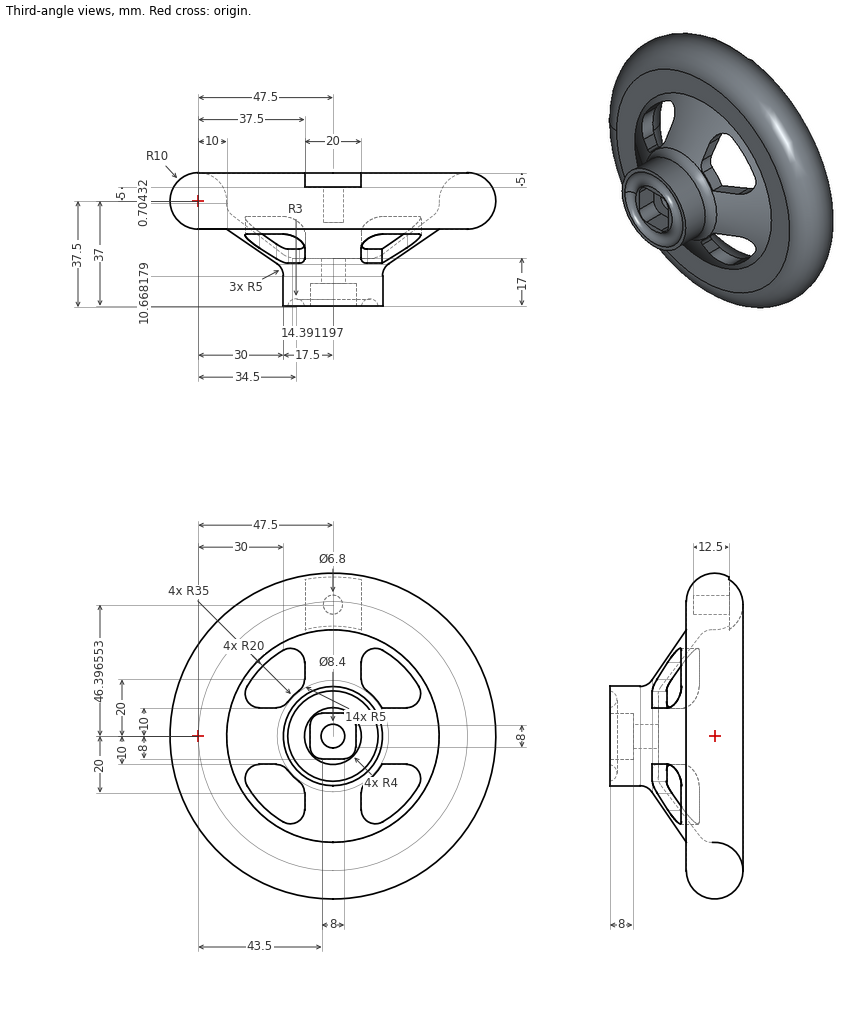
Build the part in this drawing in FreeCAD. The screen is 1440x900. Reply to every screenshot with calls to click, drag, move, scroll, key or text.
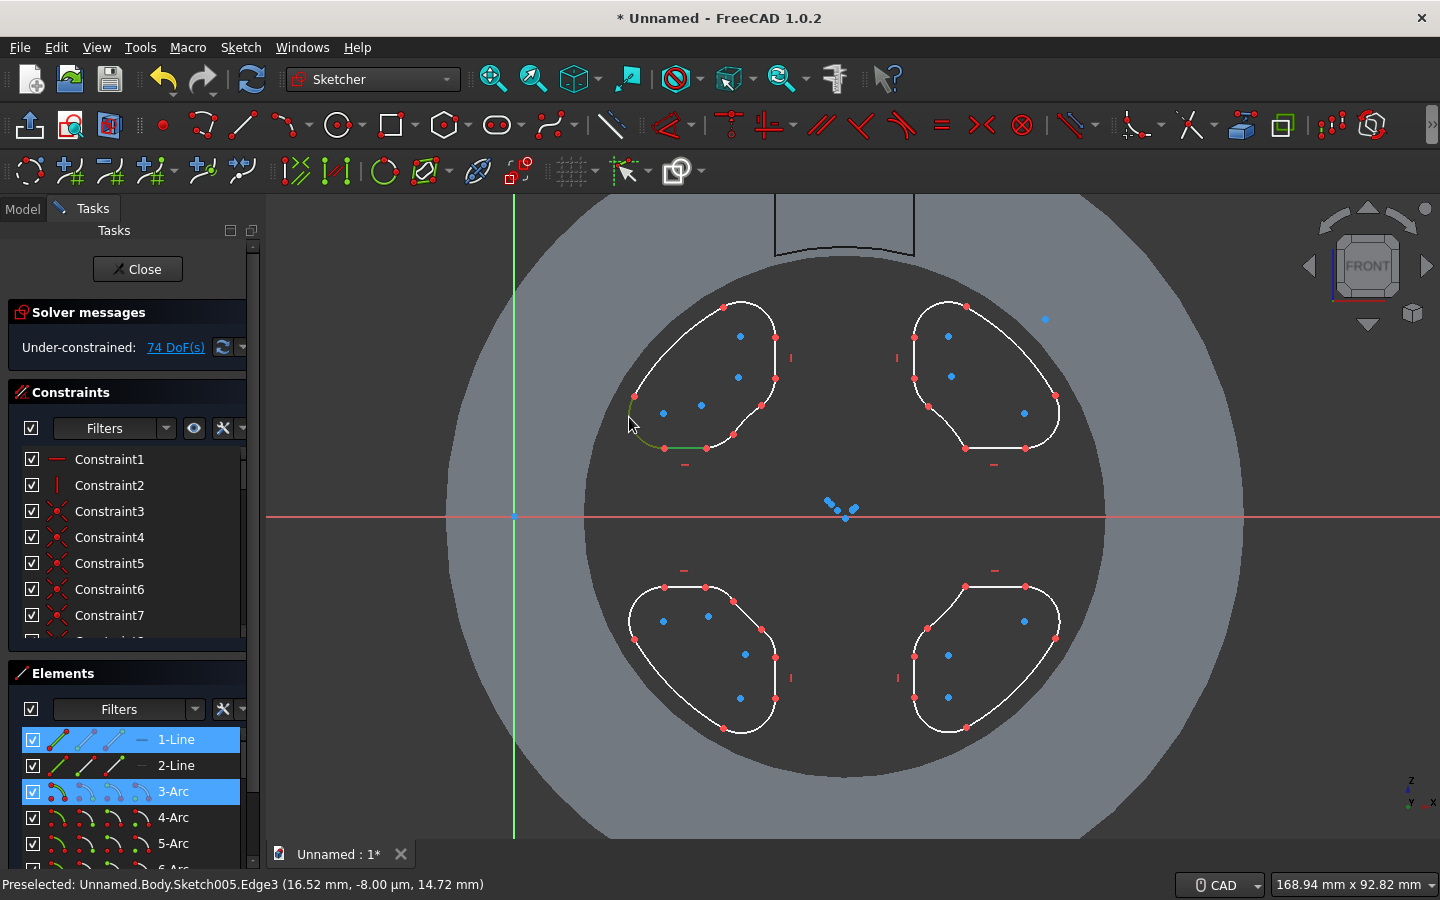
click(902, 126)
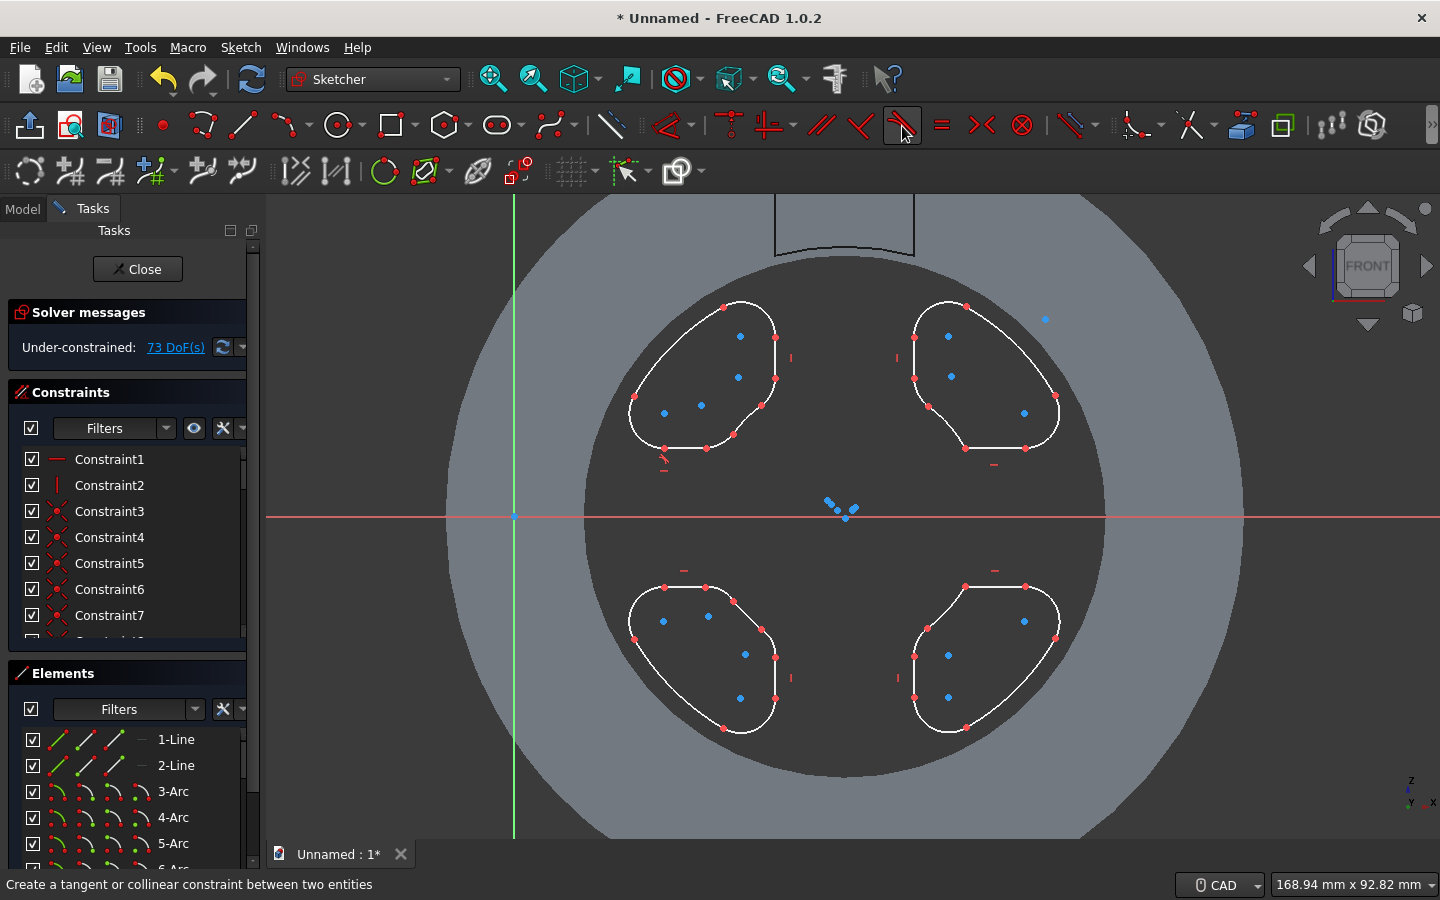
click(693, 448)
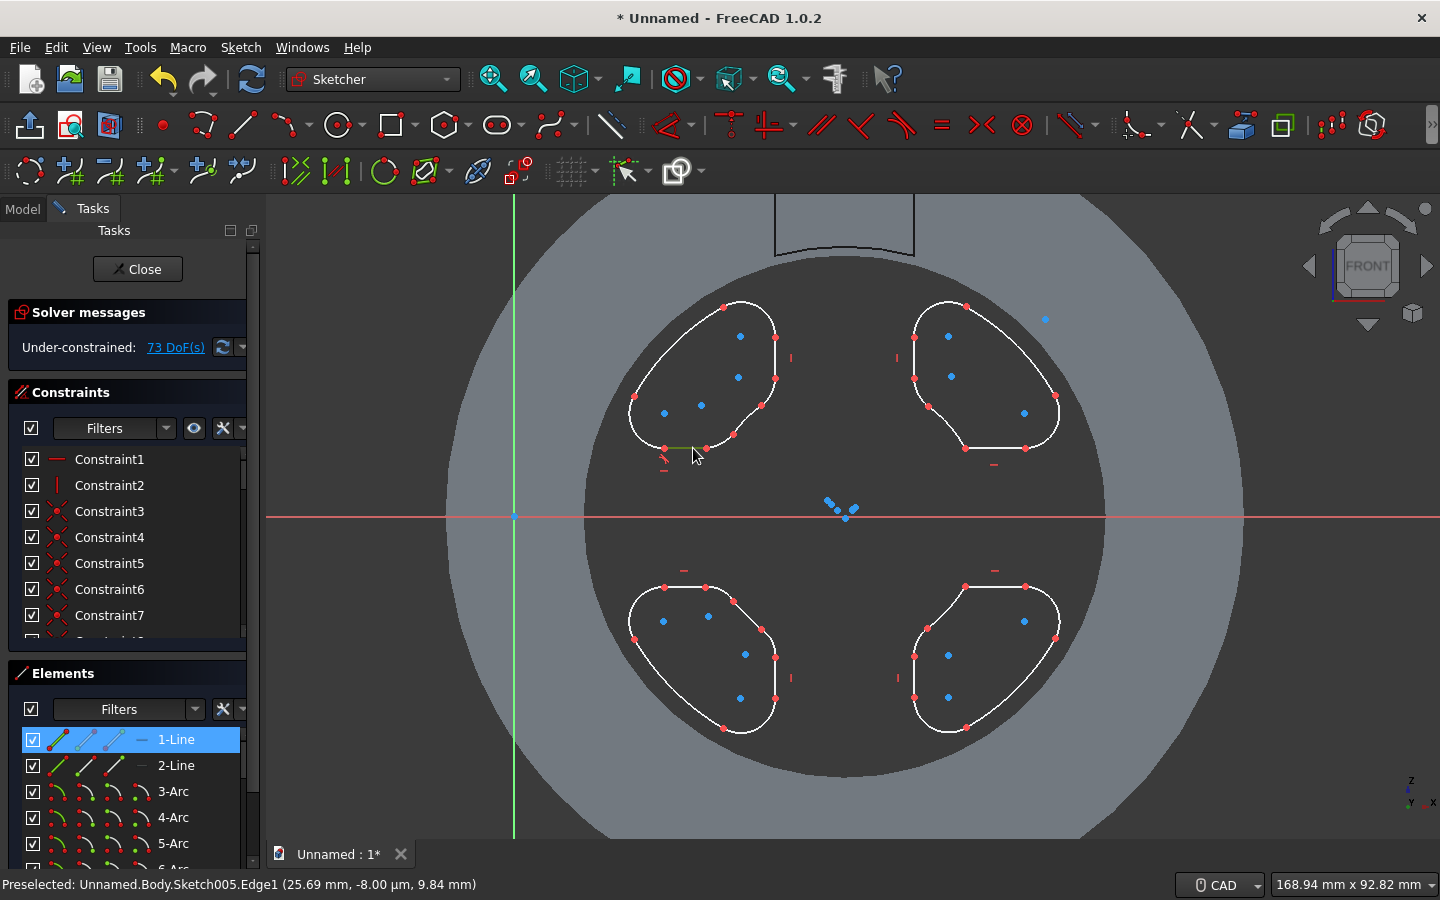
scroll(715, 446, up, 2)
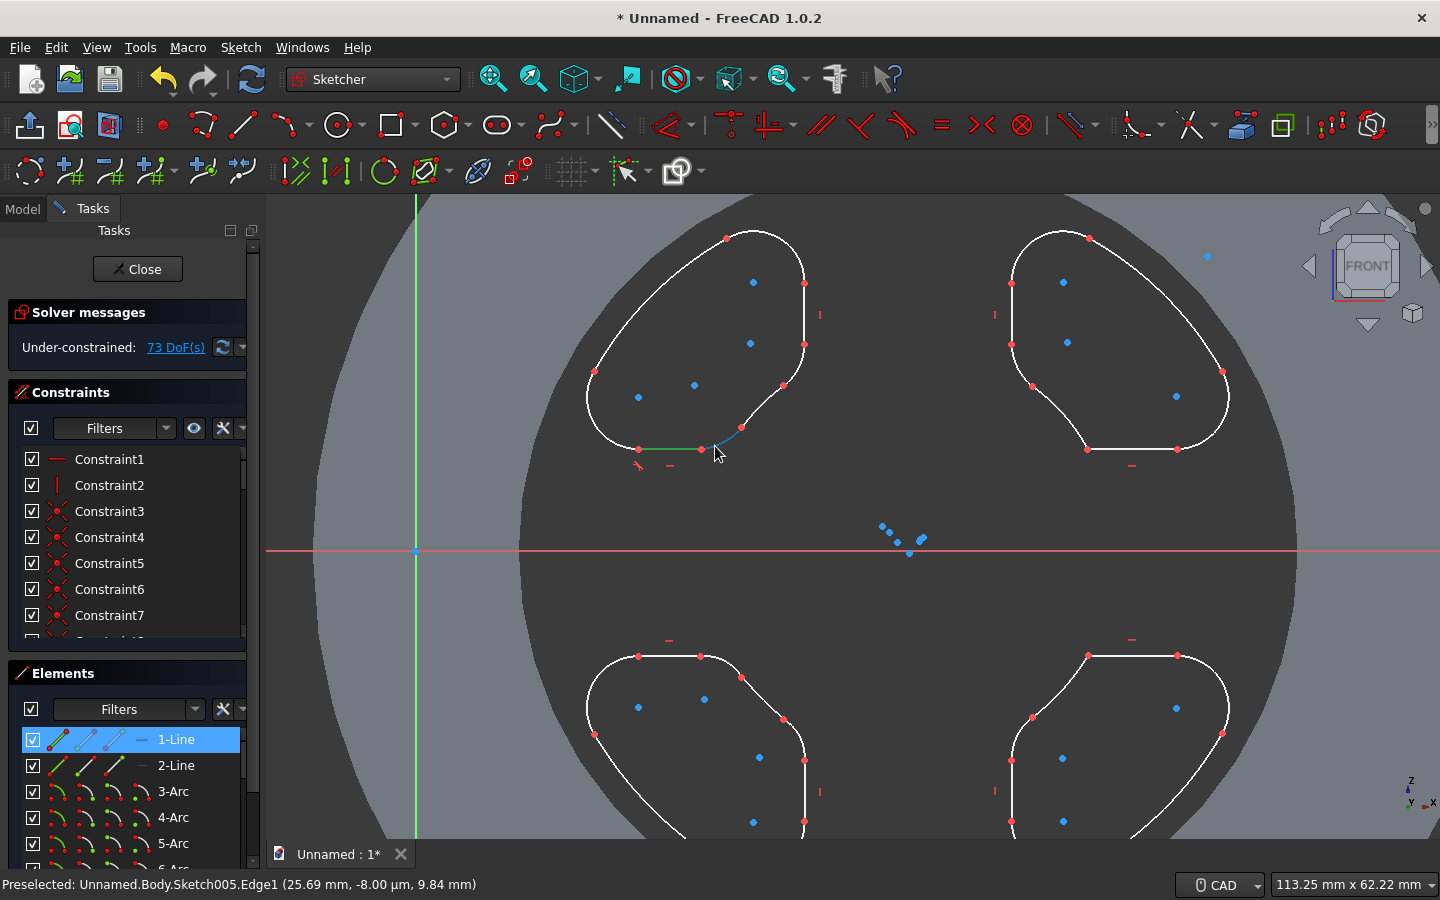
click(715, 446)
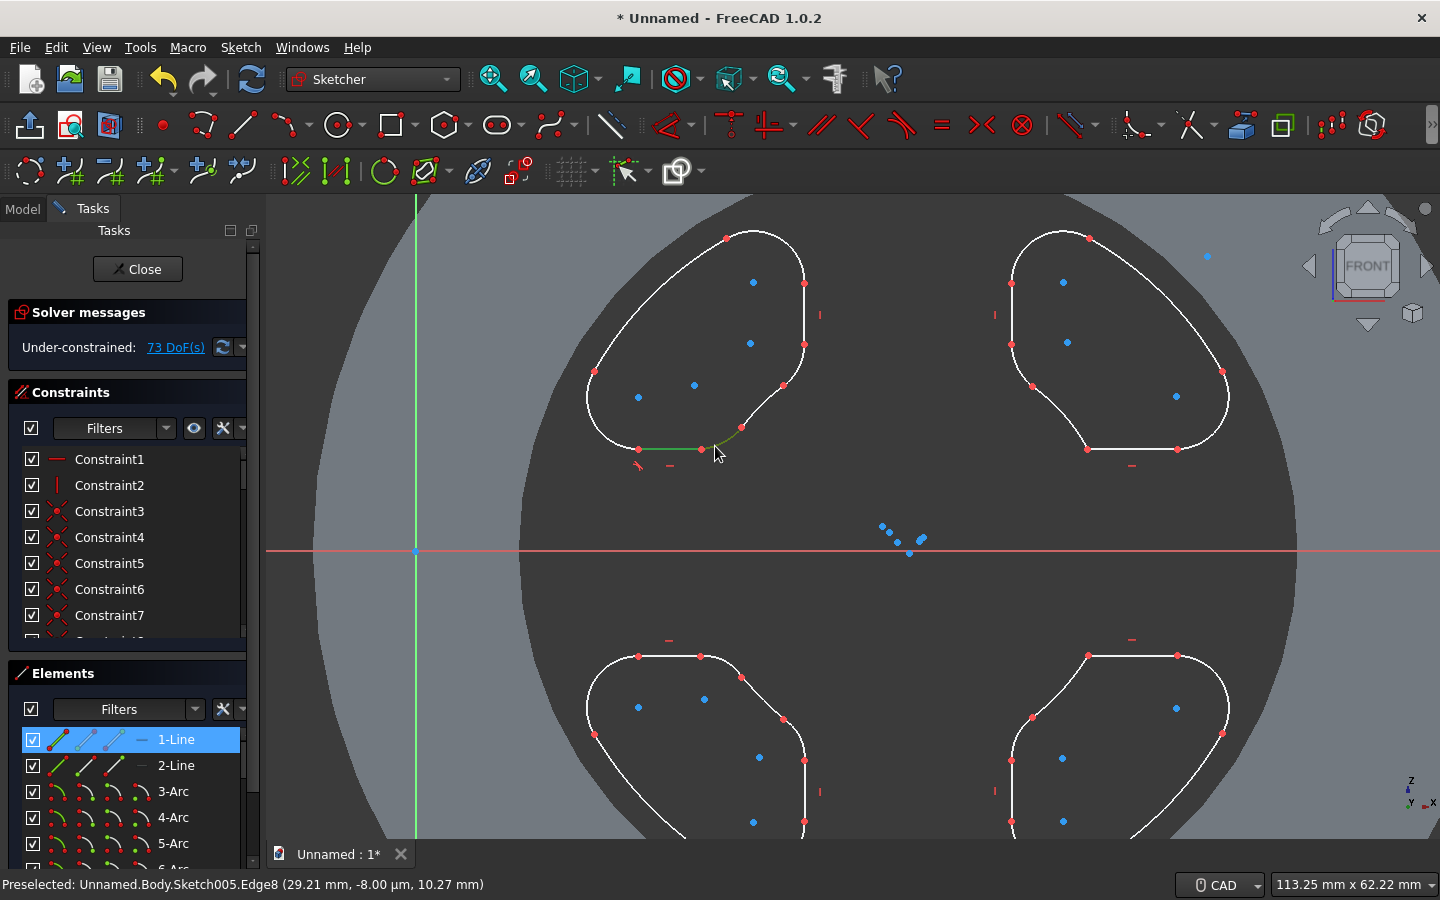
click(902, 126)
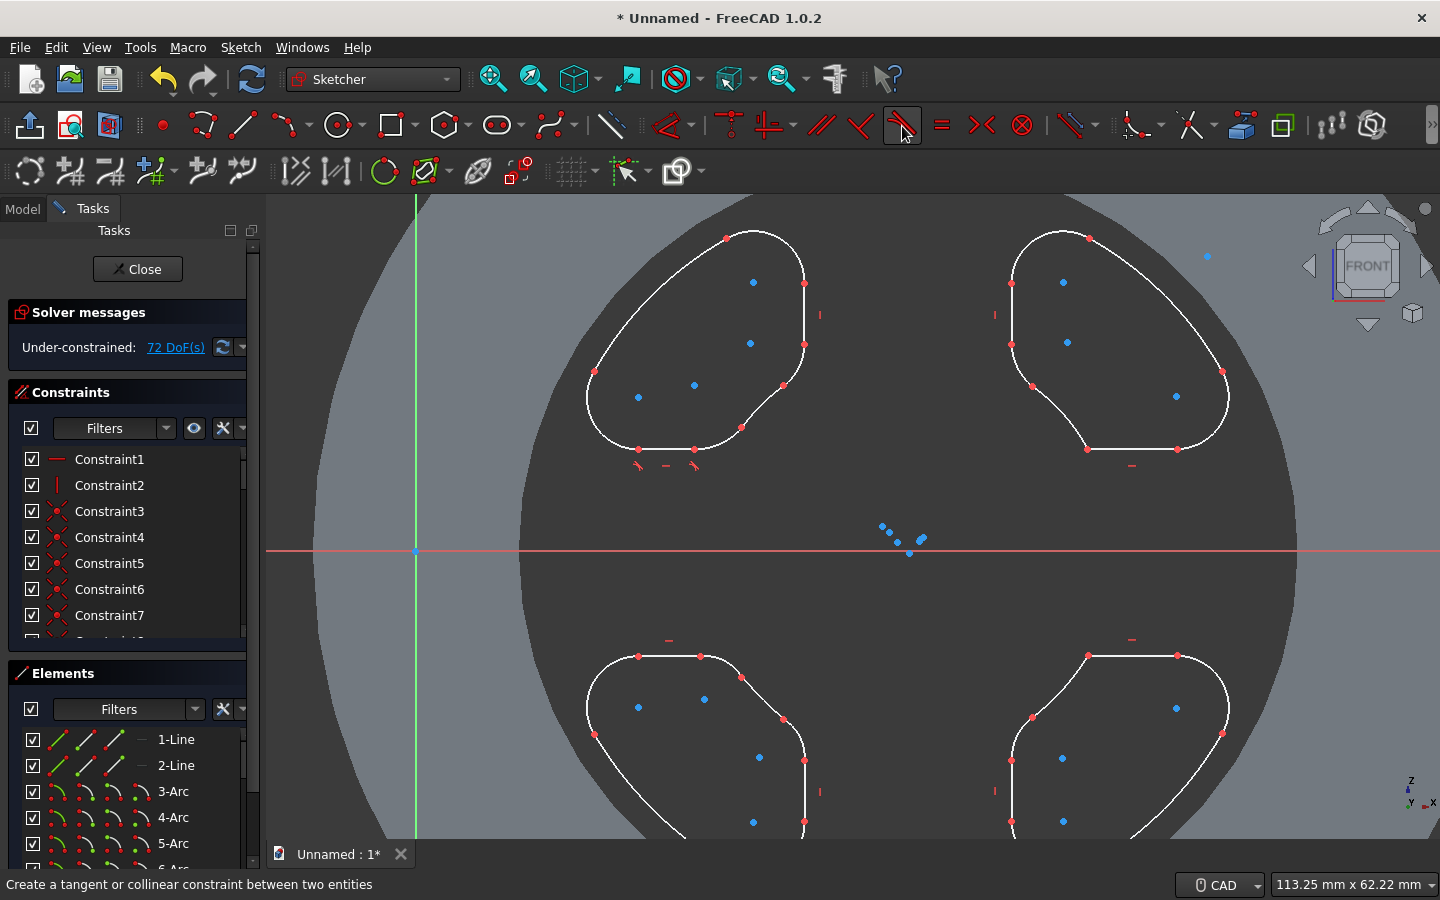
click(804, 302)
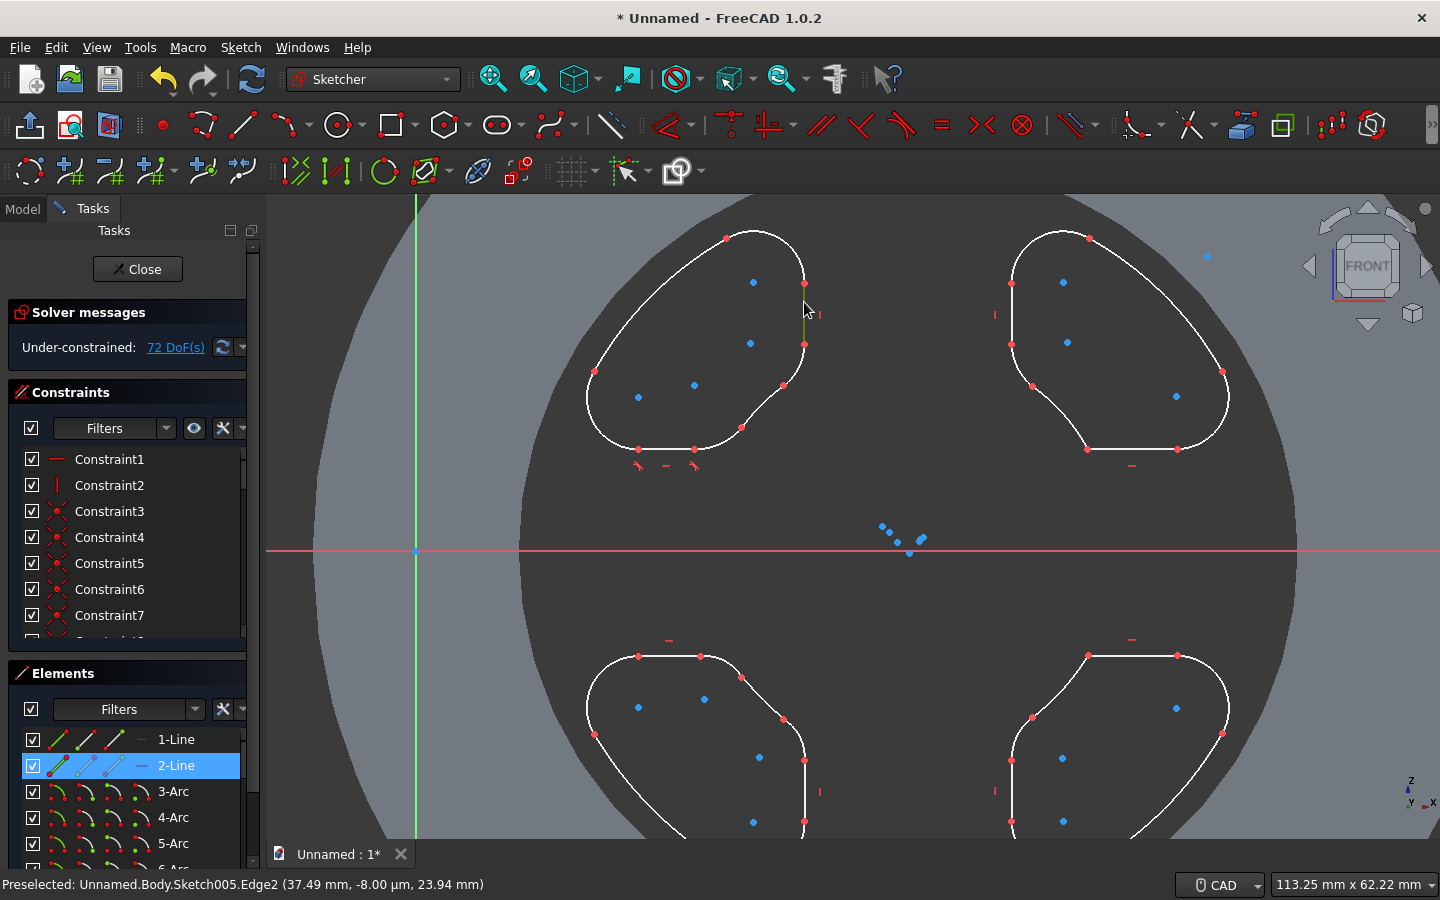
click(795, 253)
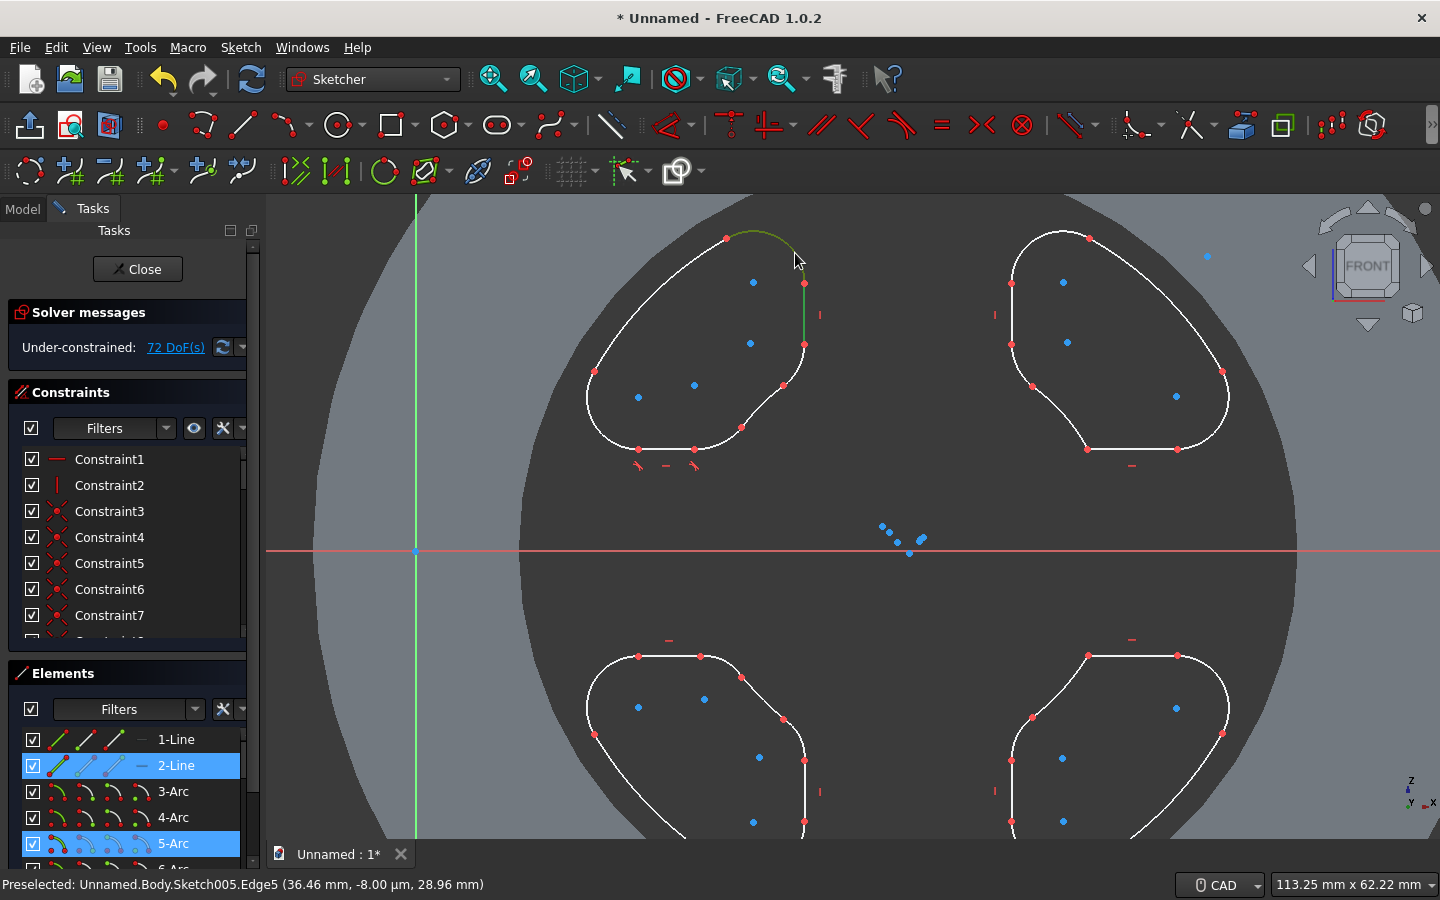
click(902, 126)